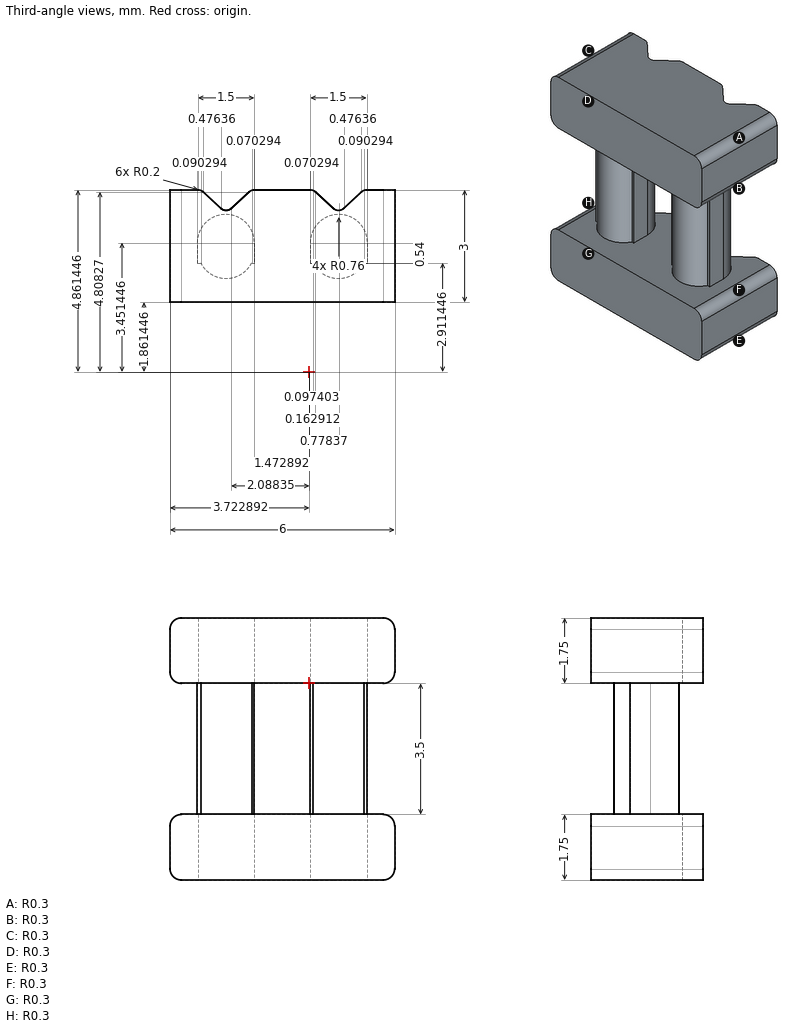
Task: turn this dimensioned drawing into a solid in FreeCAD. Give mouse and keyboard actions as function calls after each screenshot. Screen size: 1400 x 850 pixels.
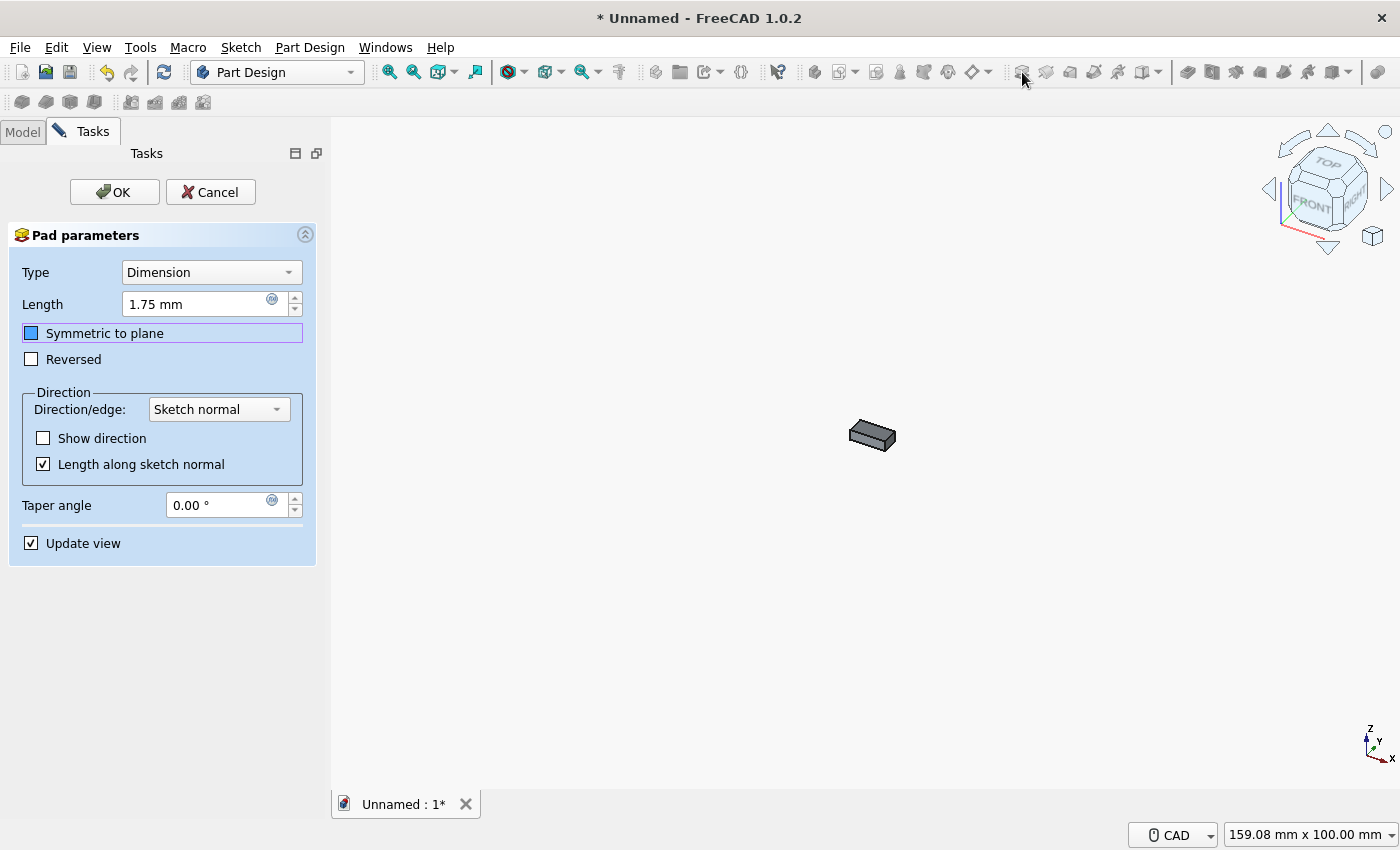
click(115, 192)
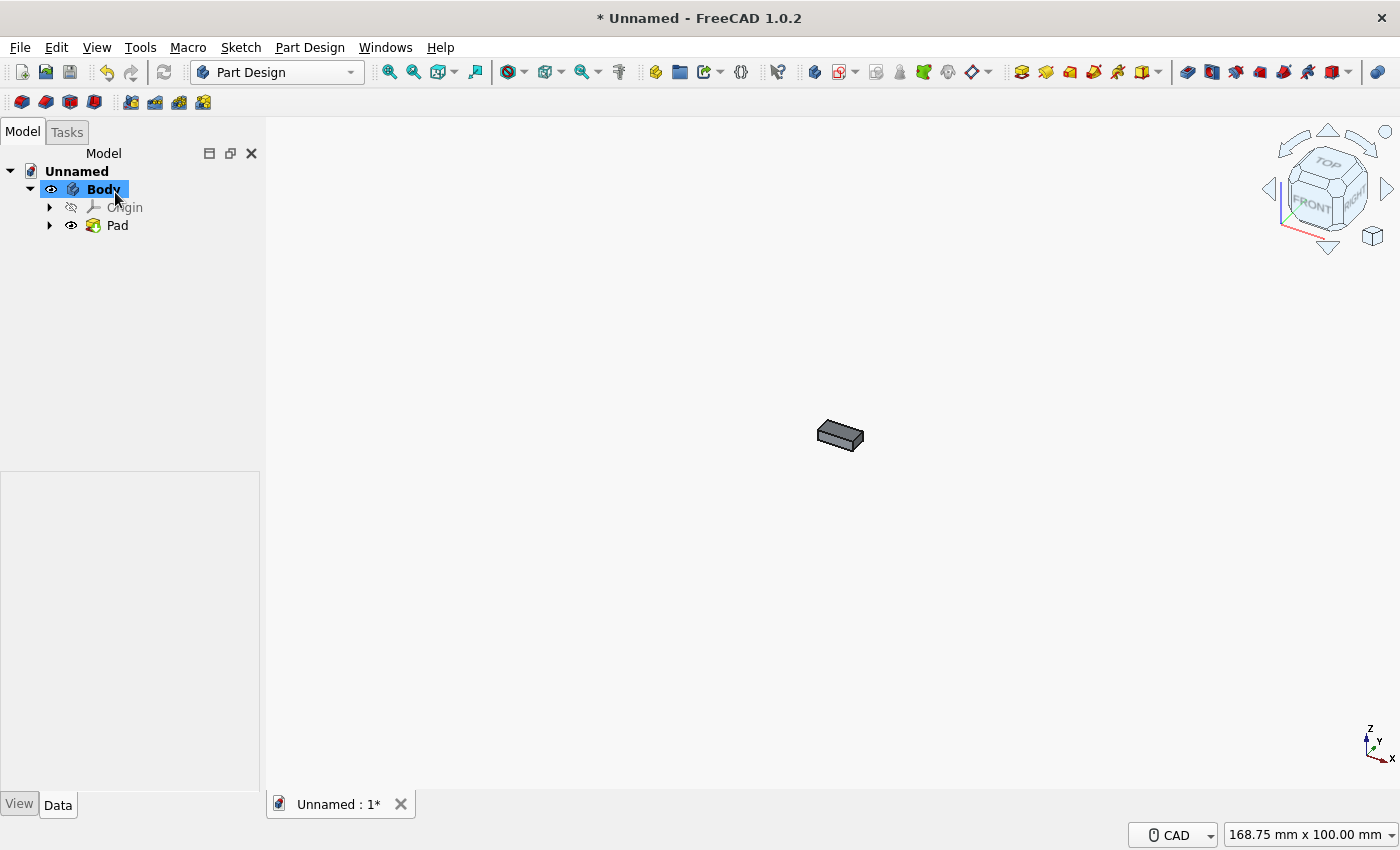
key(v)
key(f)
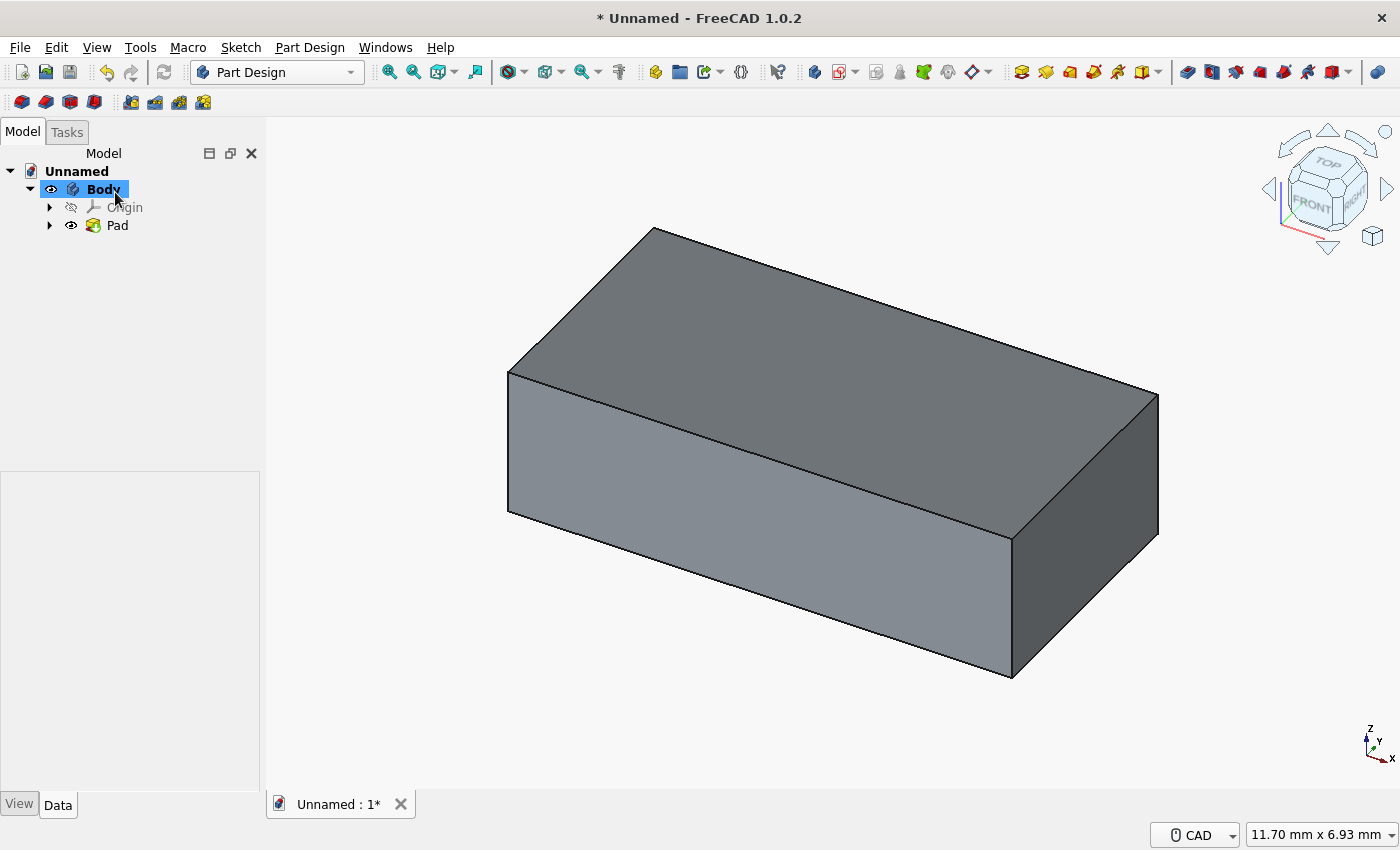
click(840, 72)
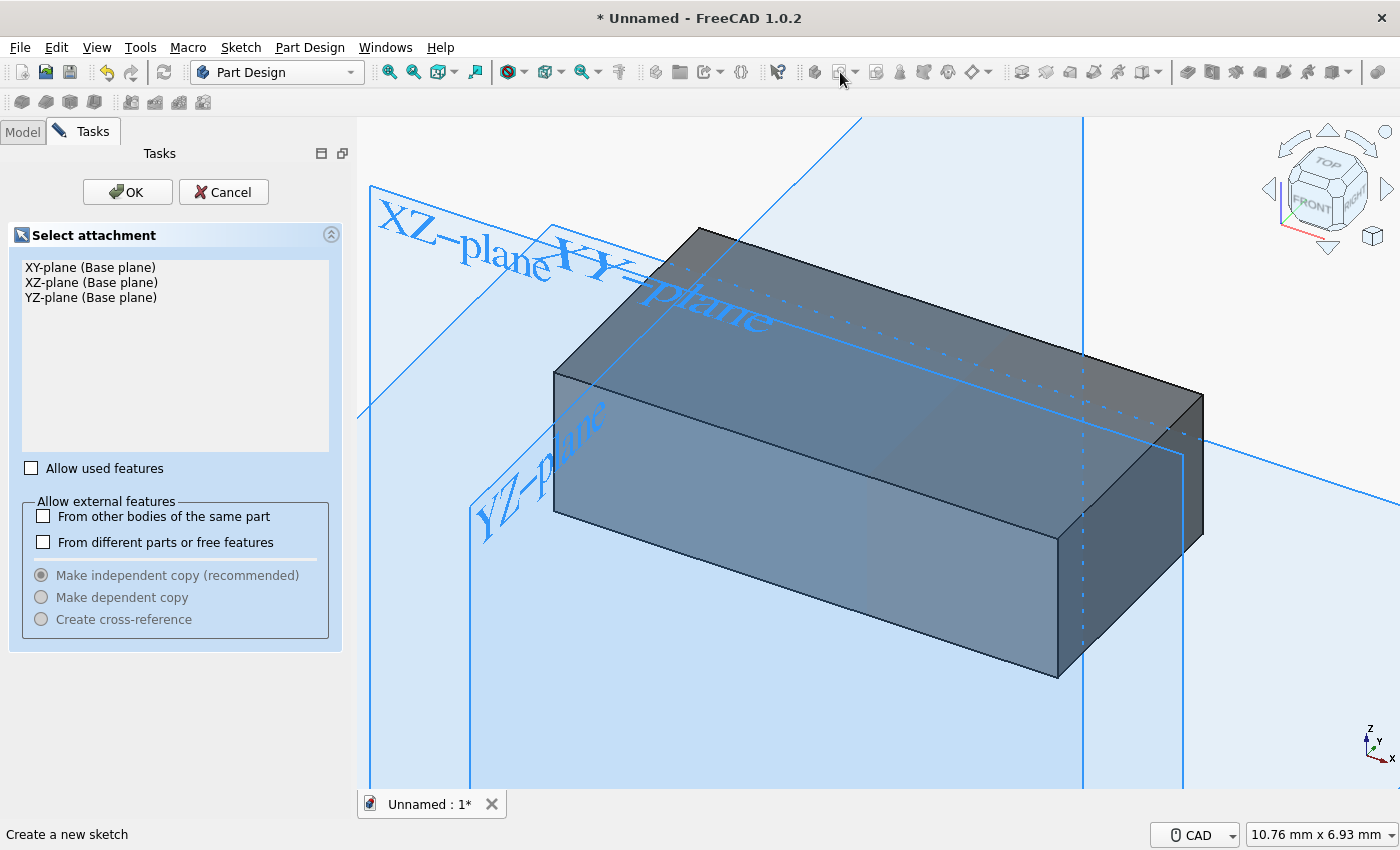
click(82, 268)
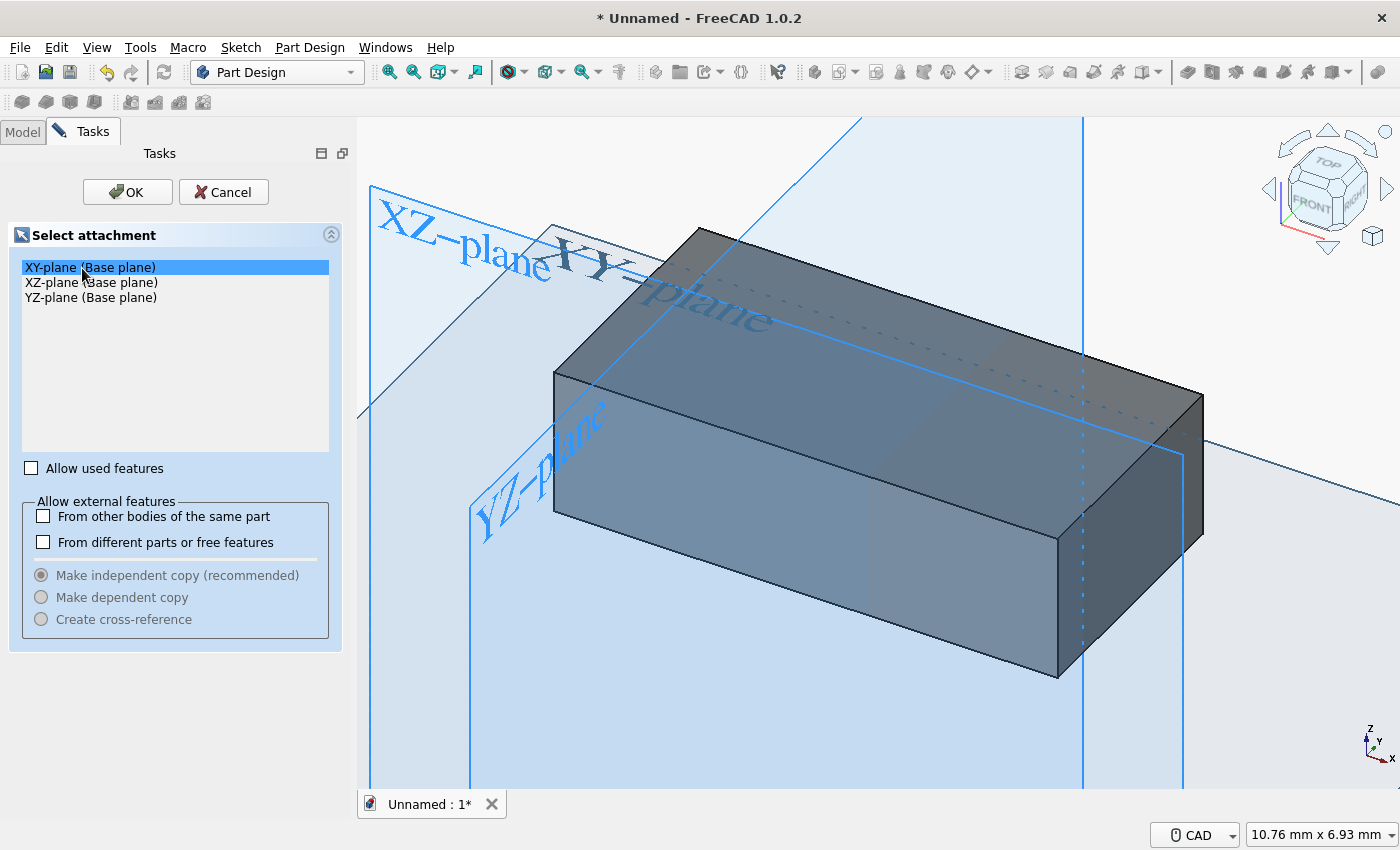
click(128, 192)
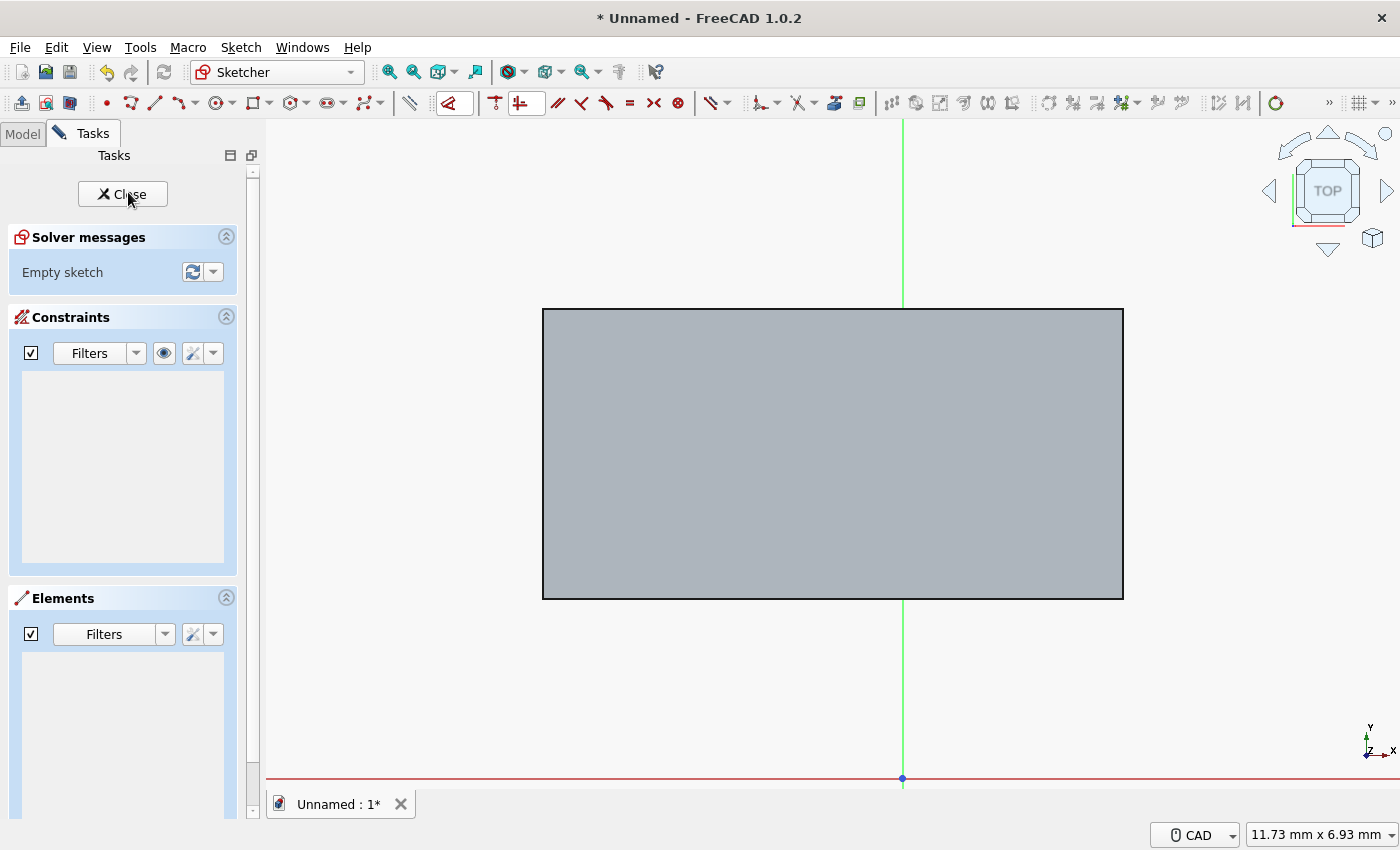
click(70, 104)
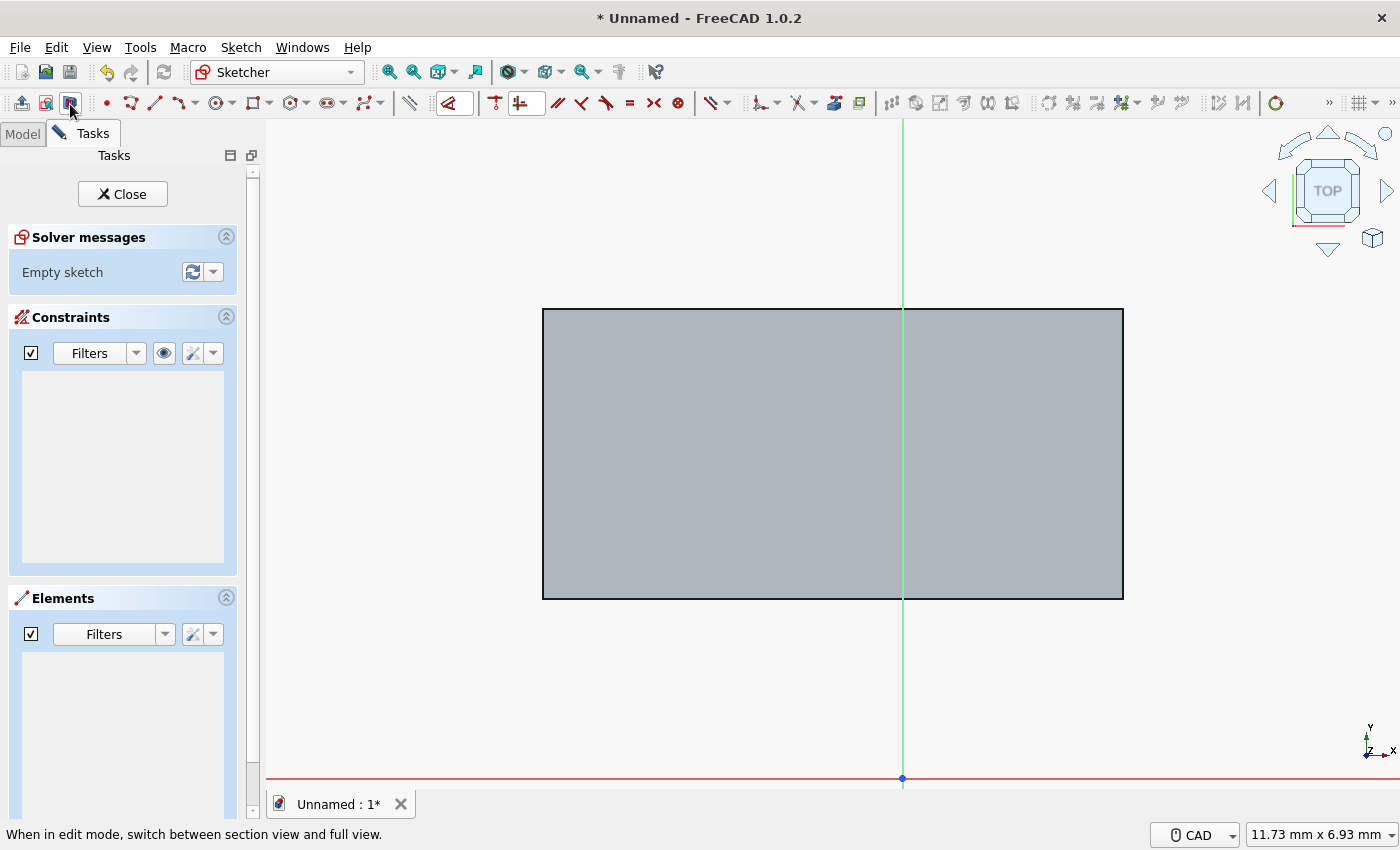
scroll(455, 147, down, 1)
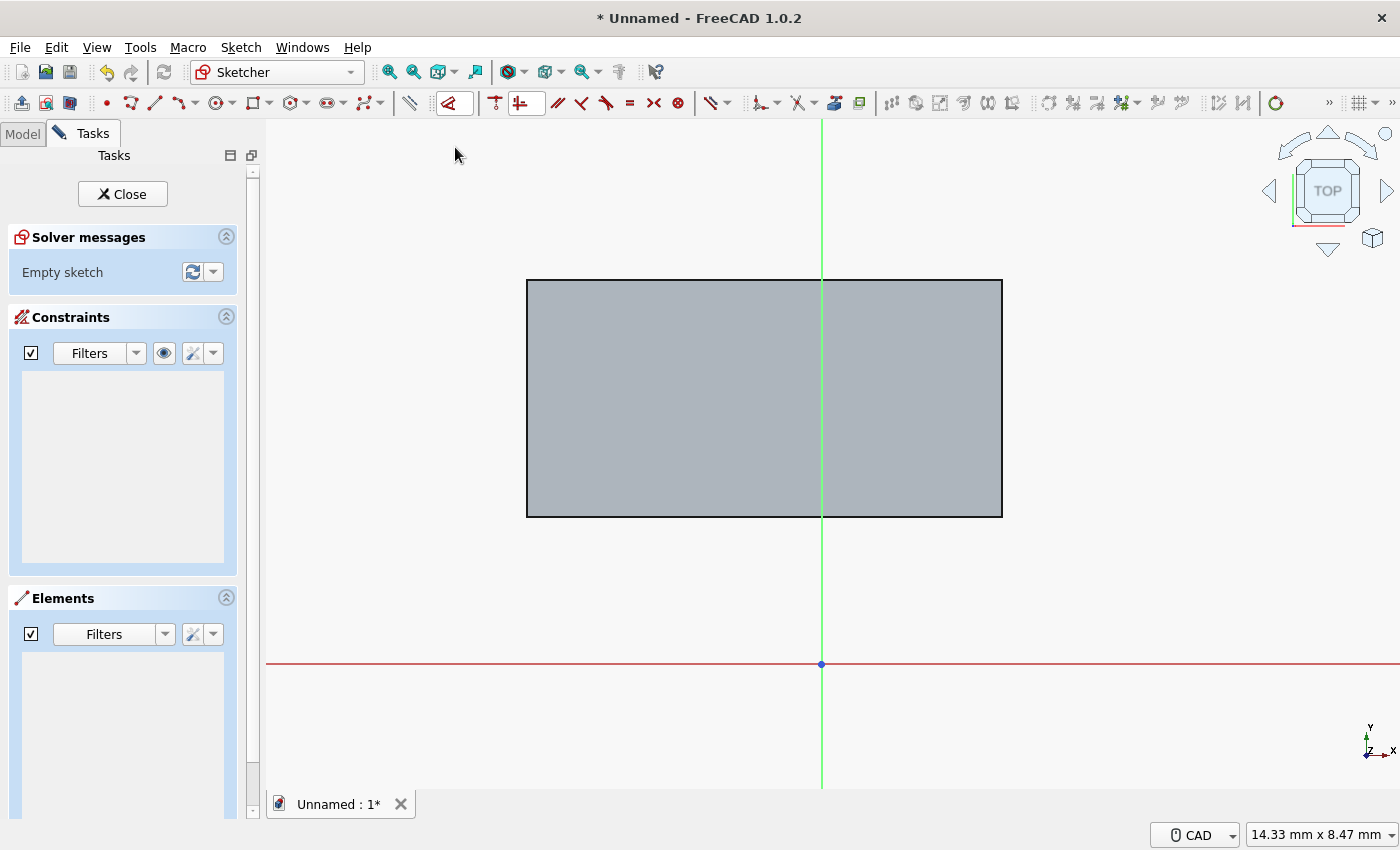
key(g)
key(m)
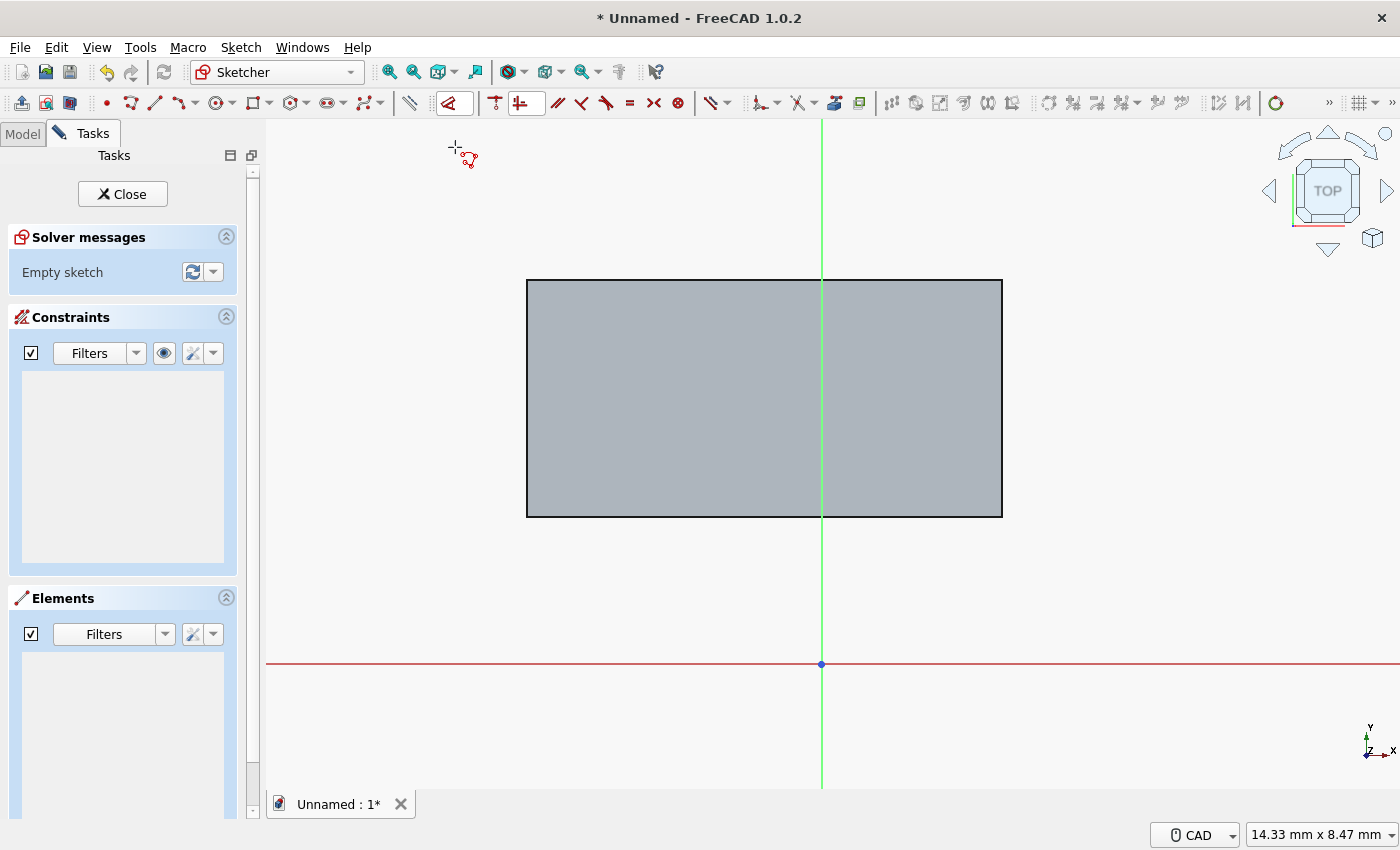
scroll(829, 434, up, 4)